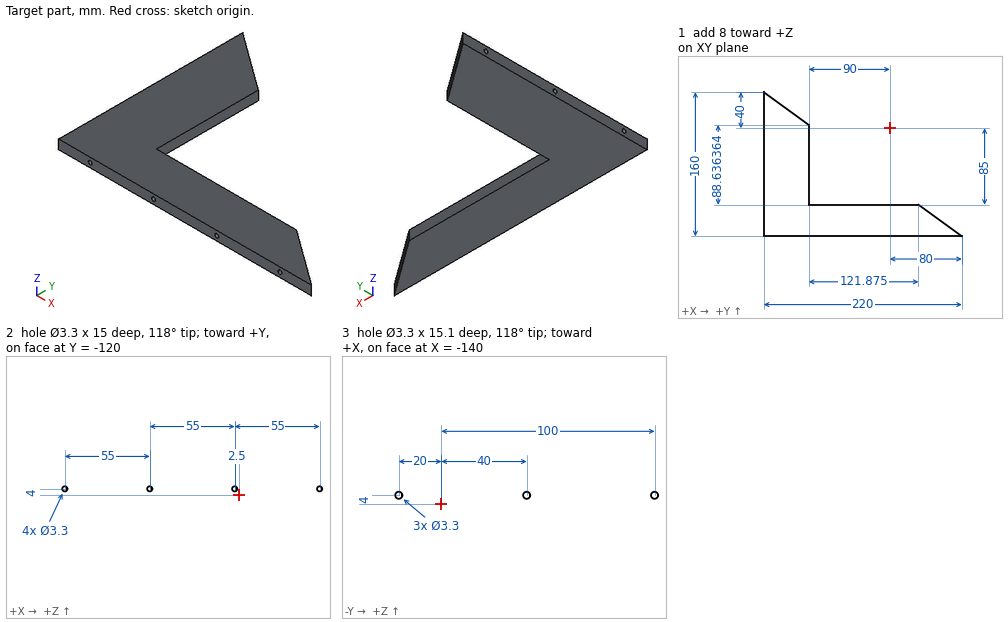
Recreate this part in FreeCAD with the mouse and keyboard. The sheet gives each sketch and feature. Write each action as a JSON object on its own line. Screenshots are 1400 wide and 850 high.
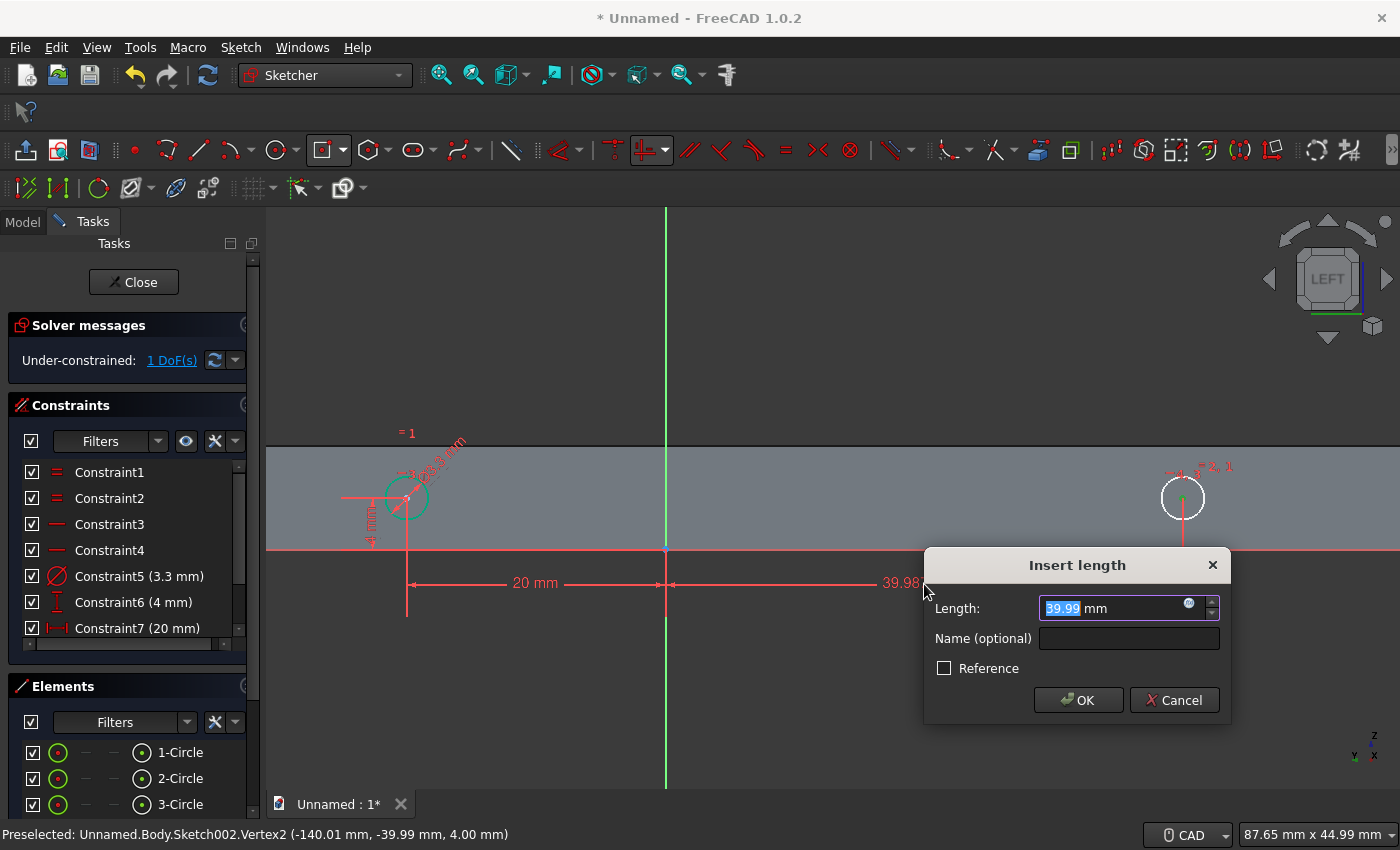
{"action": "type", "text": "40"}
{"action": "key", "text": "Return"}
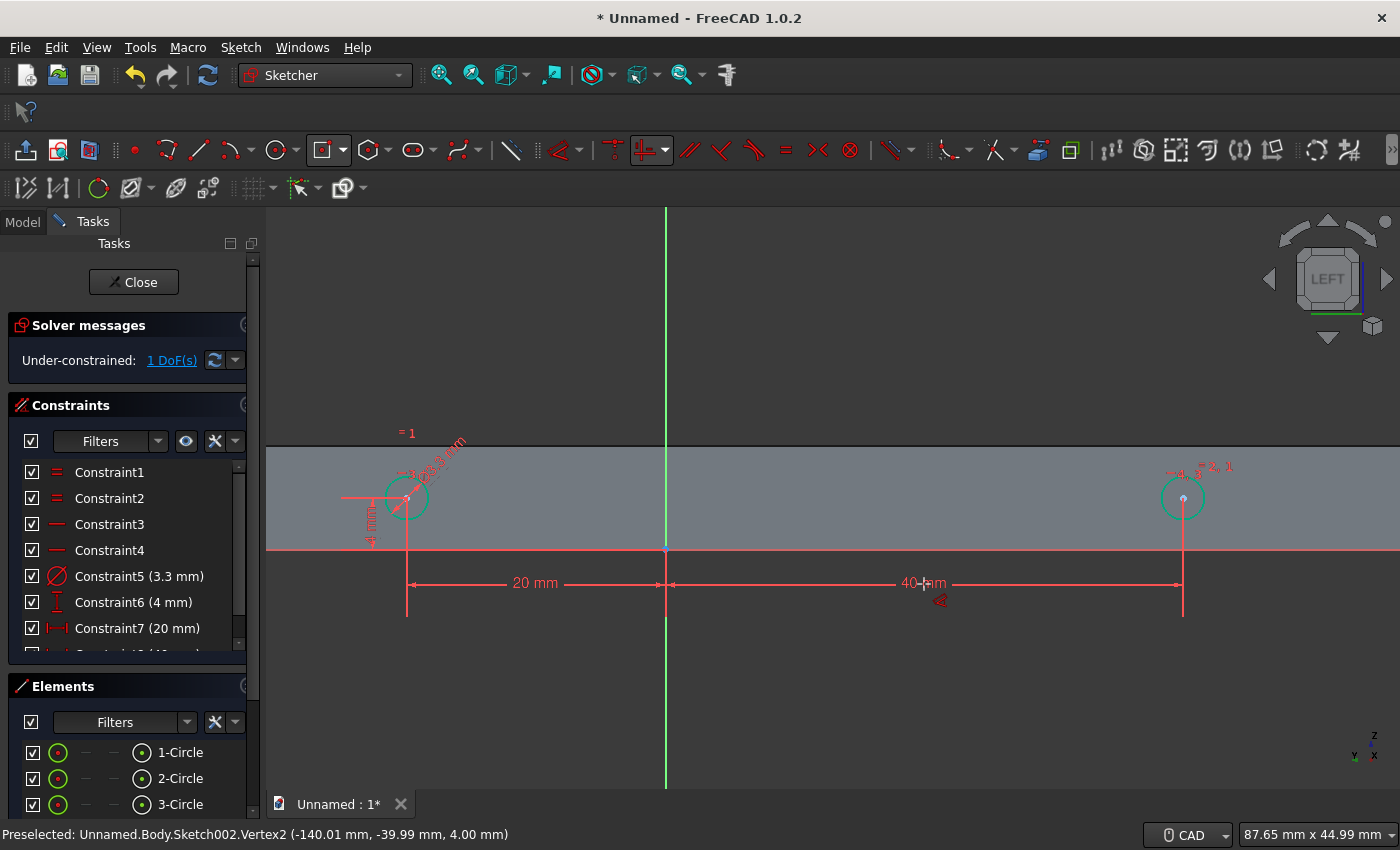
{"action": "scroll", "coordinate": [423, 485], "scroll_direction": "down", "scroll_amount": 4}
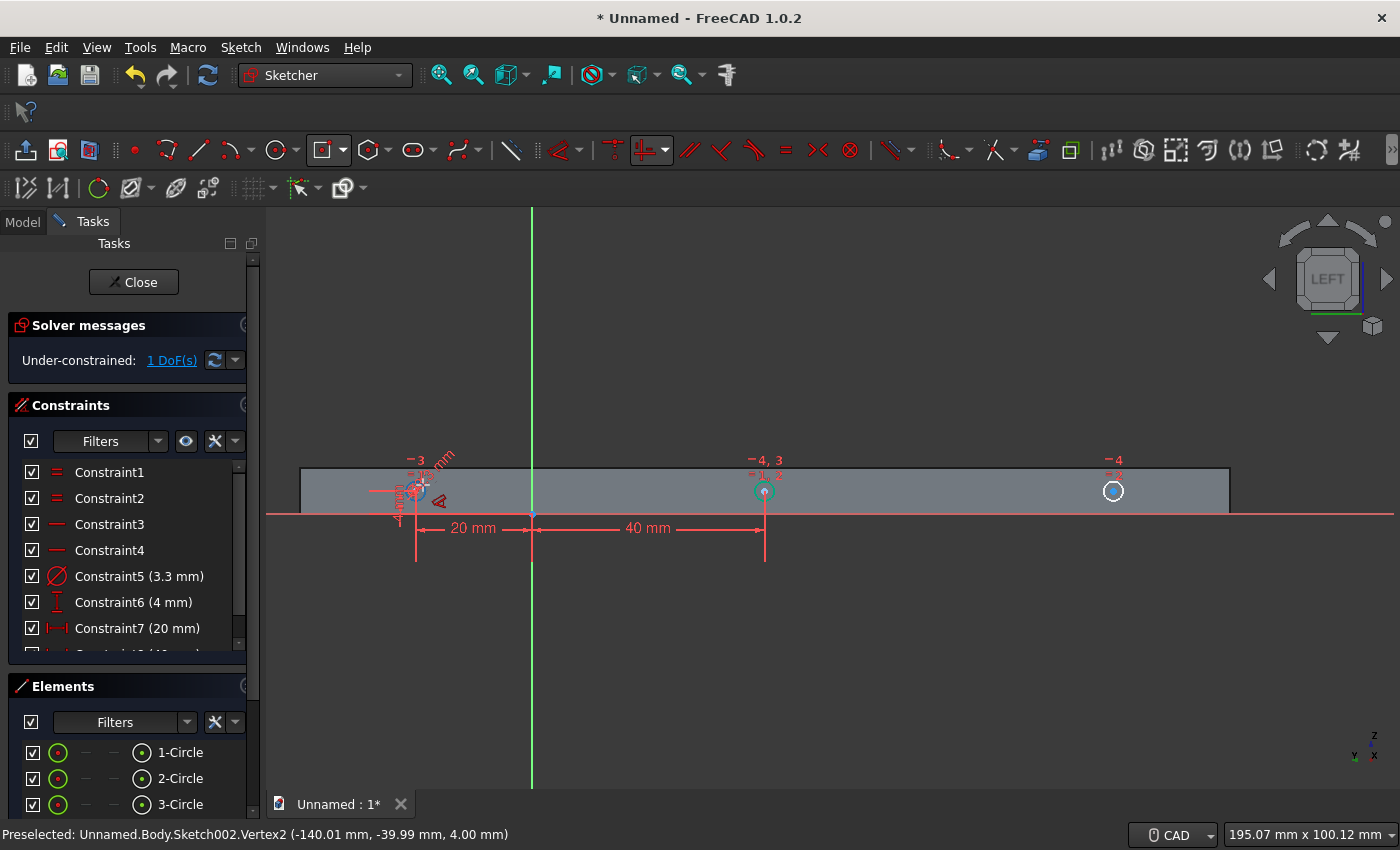
{"action": "left_click", "coordinate": [1113, 491]}
{"action": "left_click", "coordinate": [823, 548]}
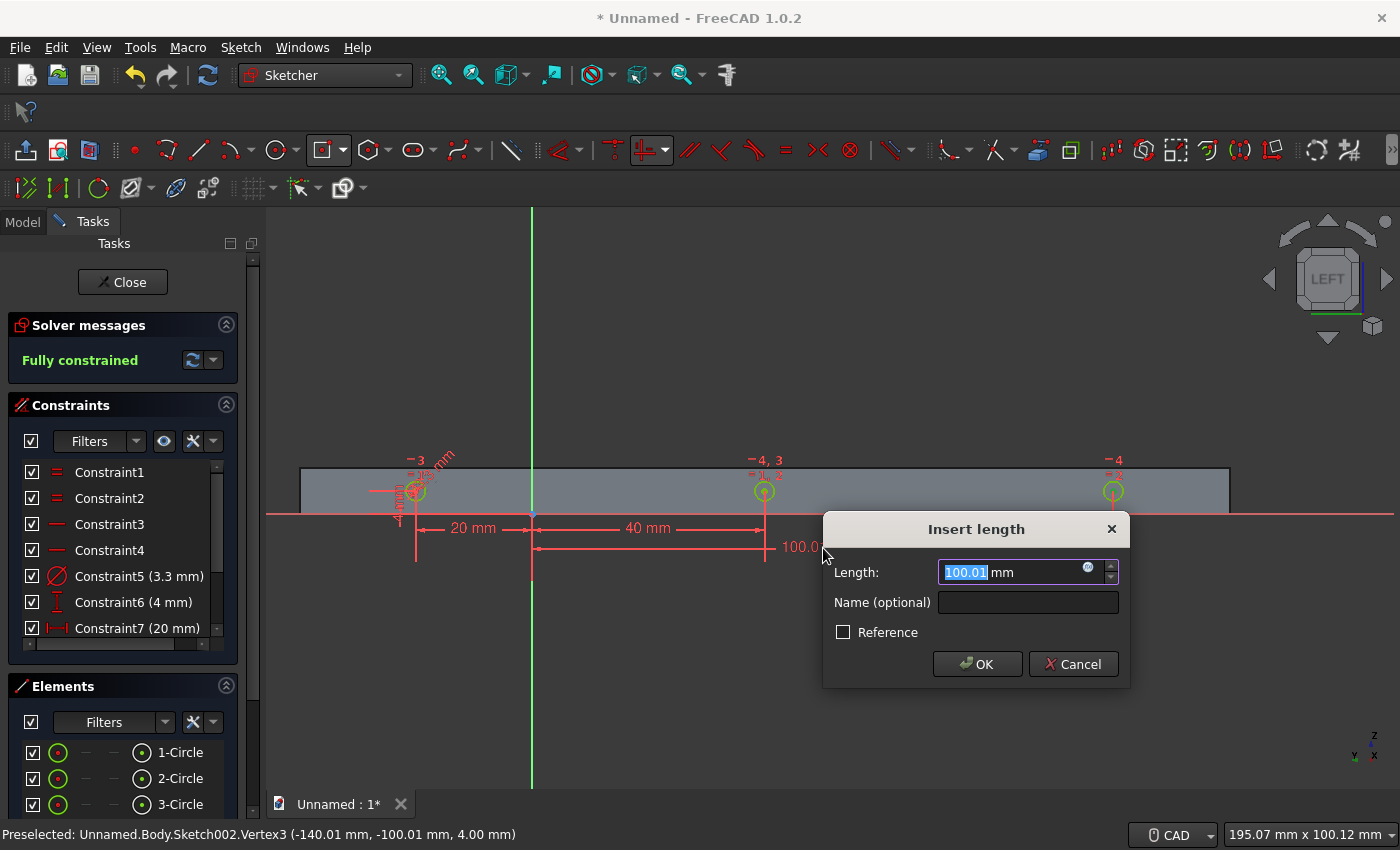
{"action": "type", "text": "100"}
{"action": "key", "text": "Return"}
{"action": "key", "text": "Escape"}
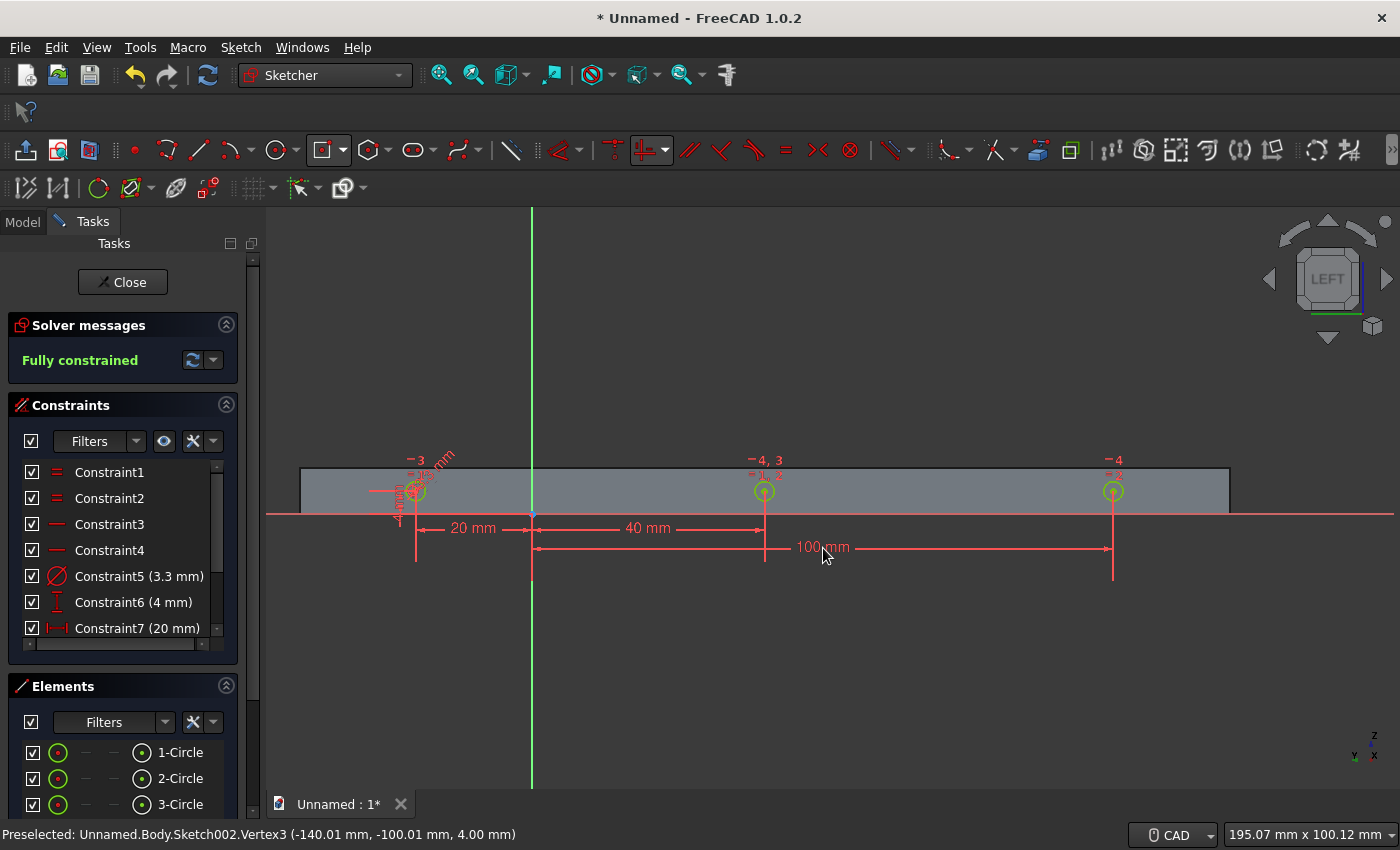
{"action": "left_click", "coordinate": [123, 282]}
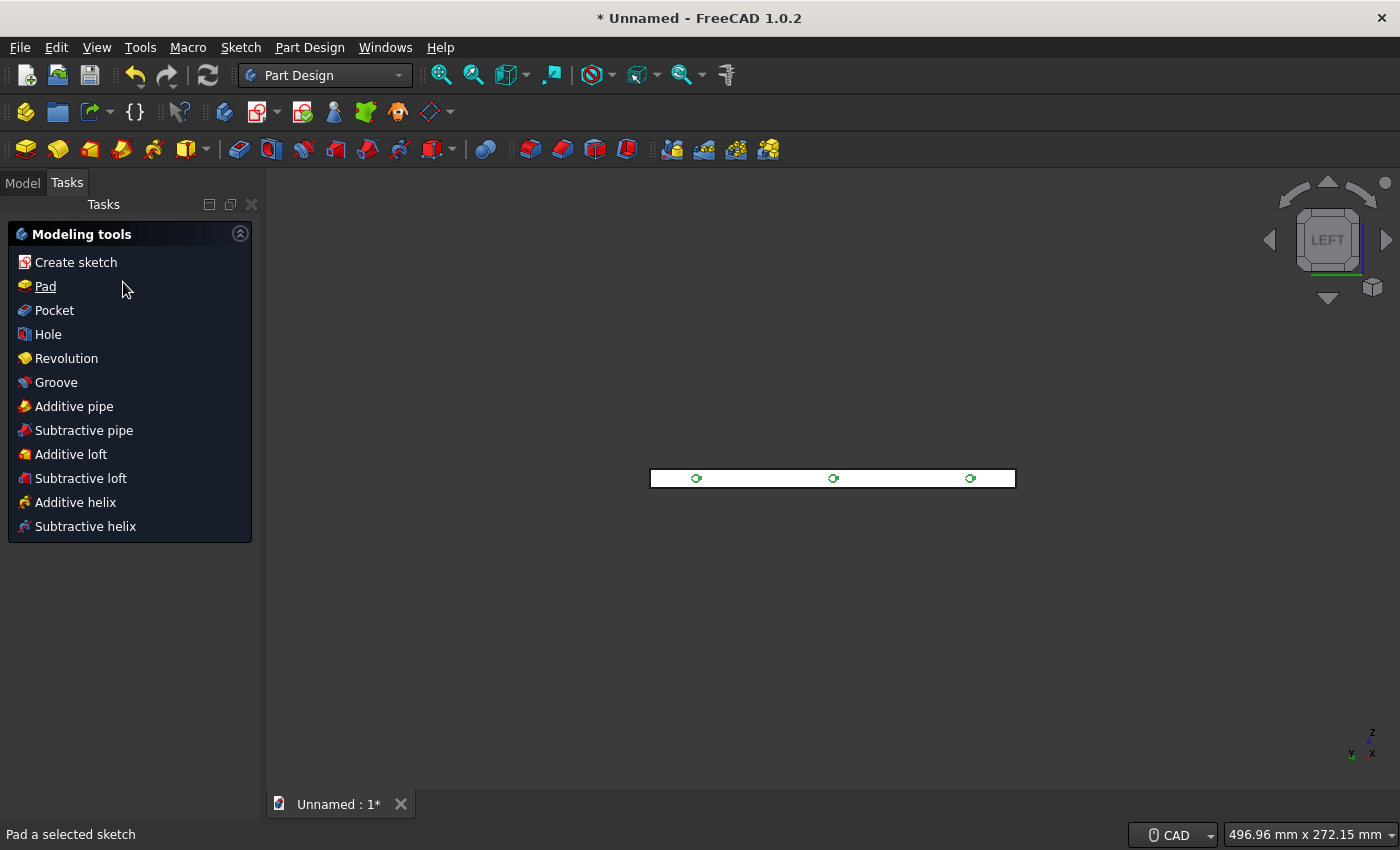
{"action": "left_click", "coordinate": [272, 150]}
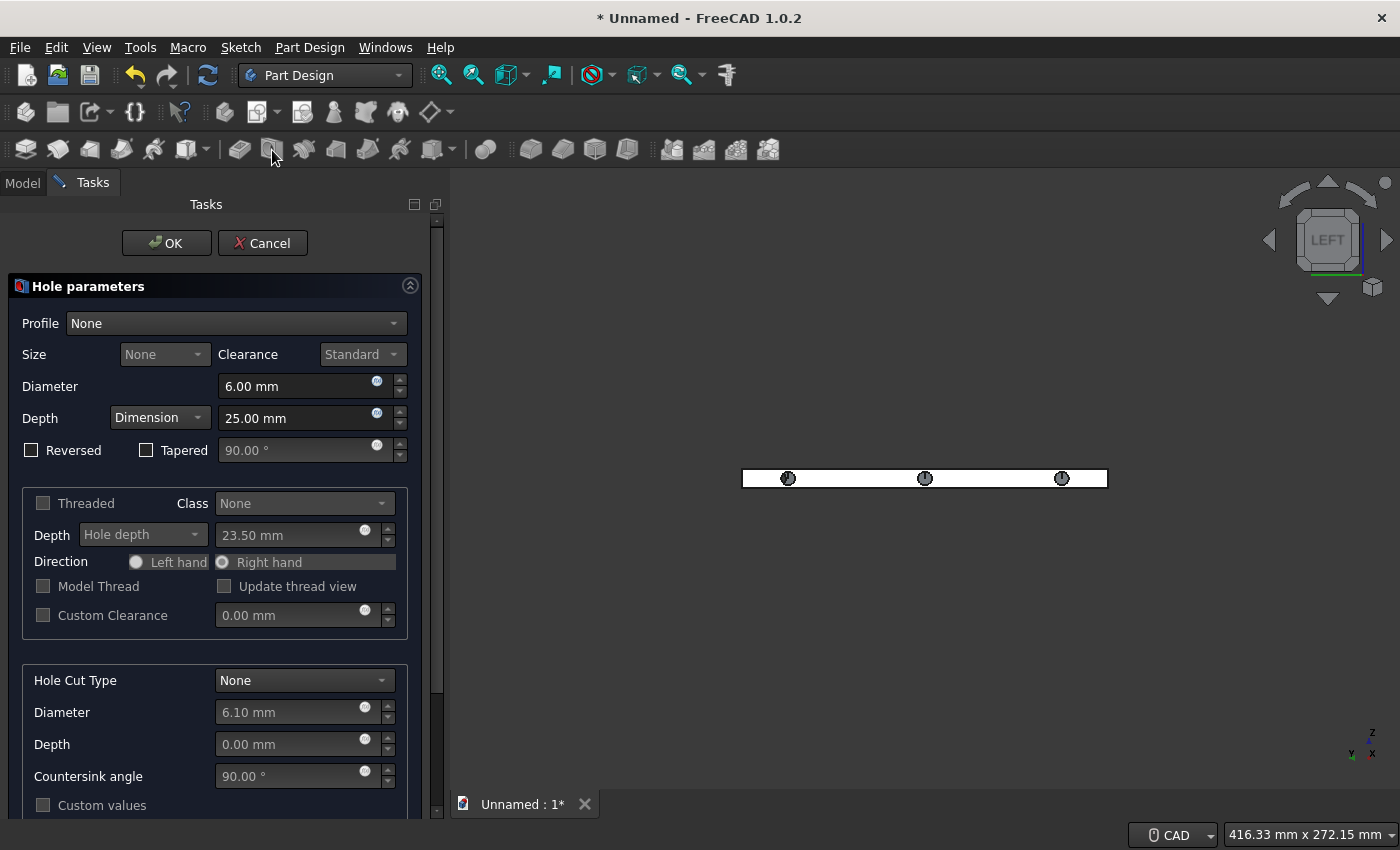
{"action": "triple_click", "coordinate": [305, 386]}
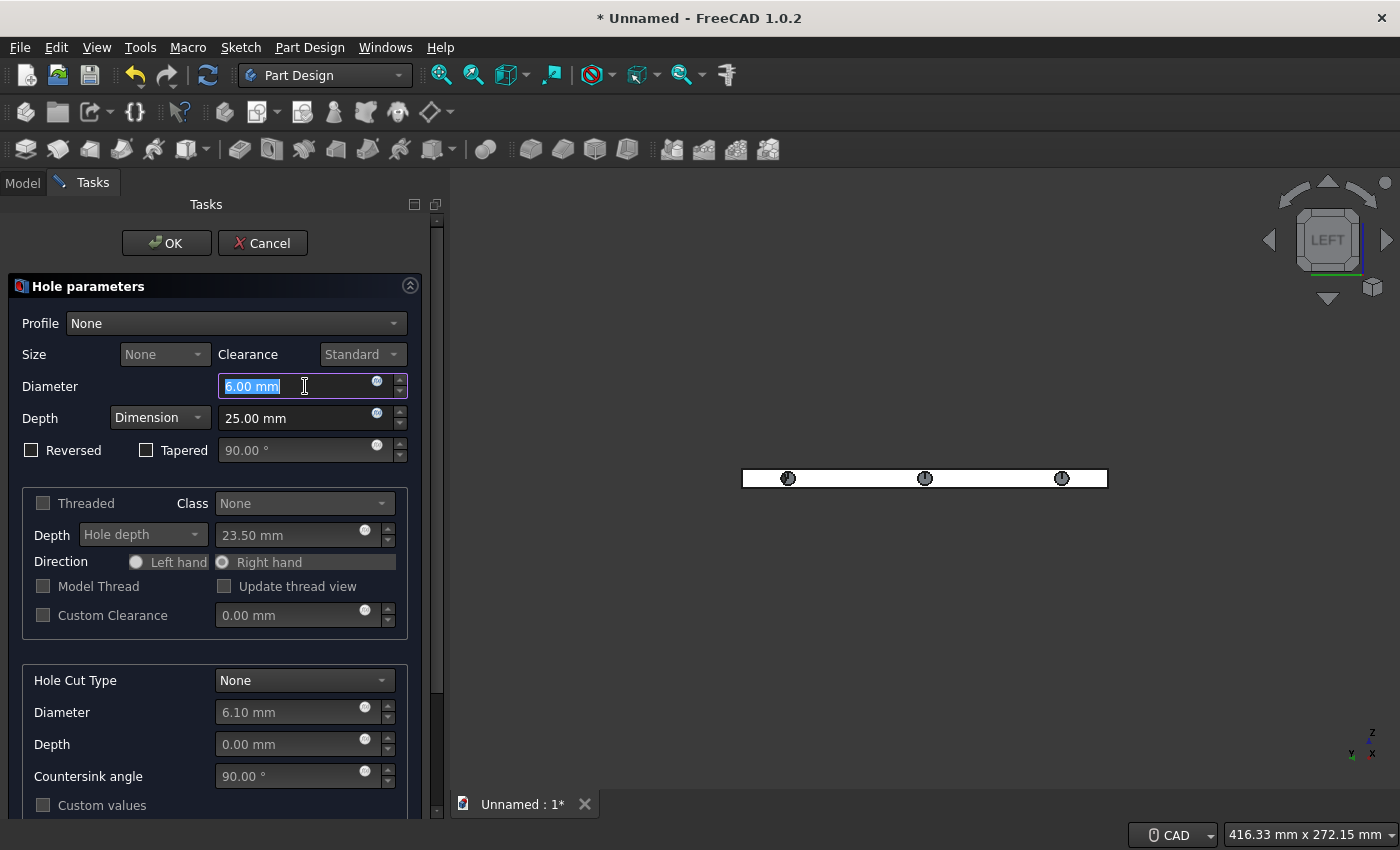
{"action": "type", "text": "3.3"}
{"action": "key", "text": "Tab"}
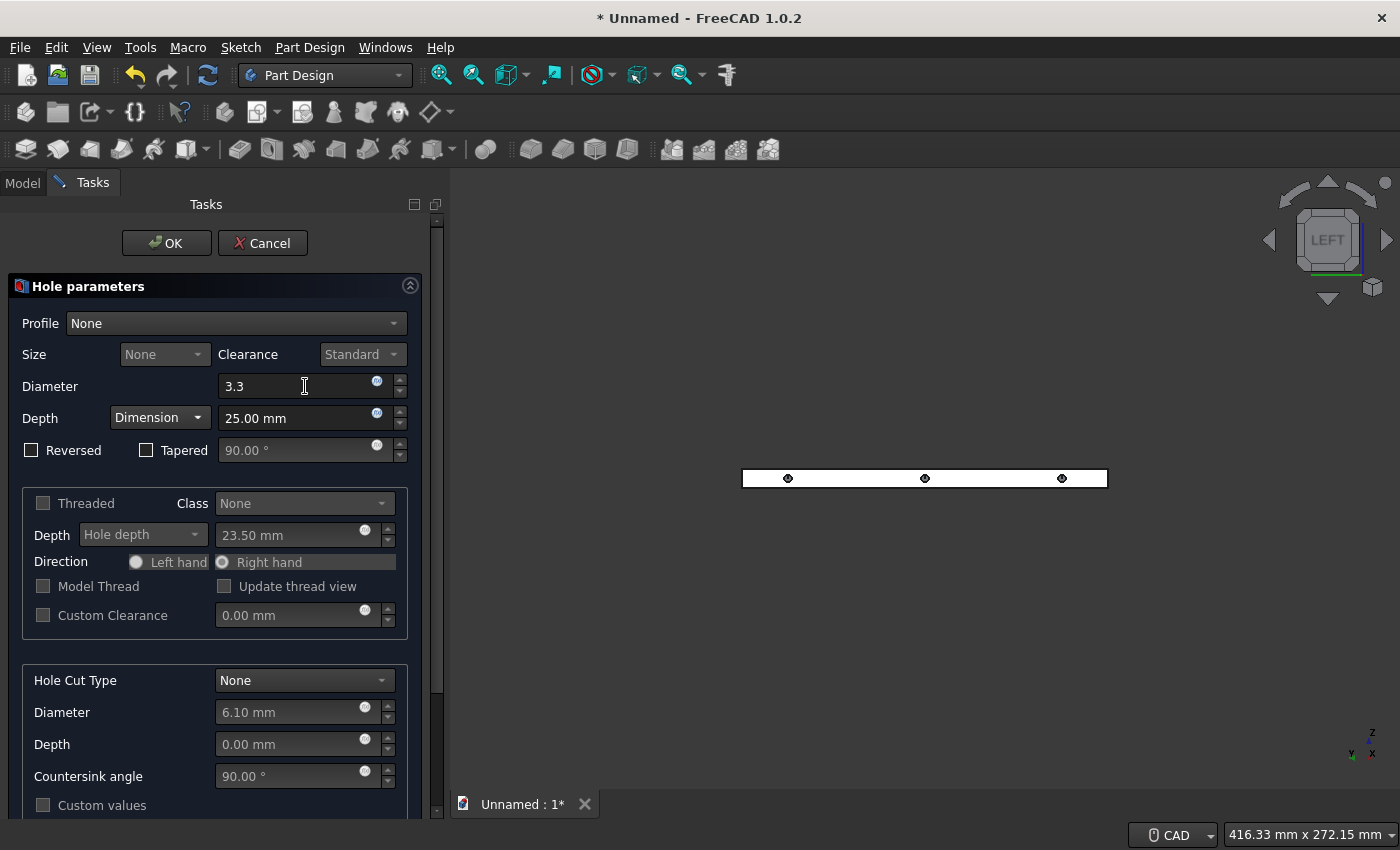
{"action": "triple_click", "coordinate": [305, 418]}